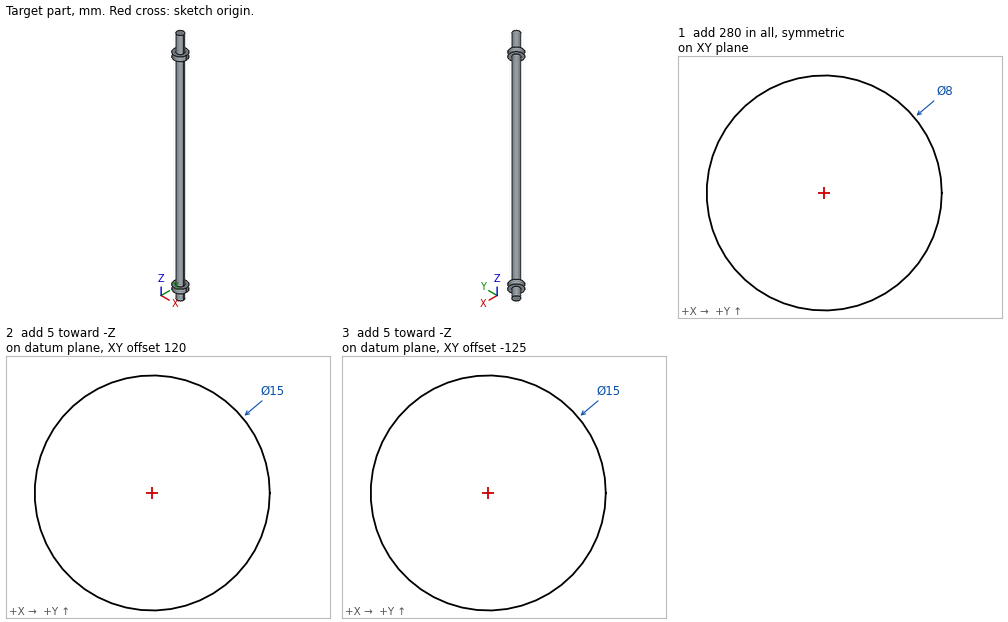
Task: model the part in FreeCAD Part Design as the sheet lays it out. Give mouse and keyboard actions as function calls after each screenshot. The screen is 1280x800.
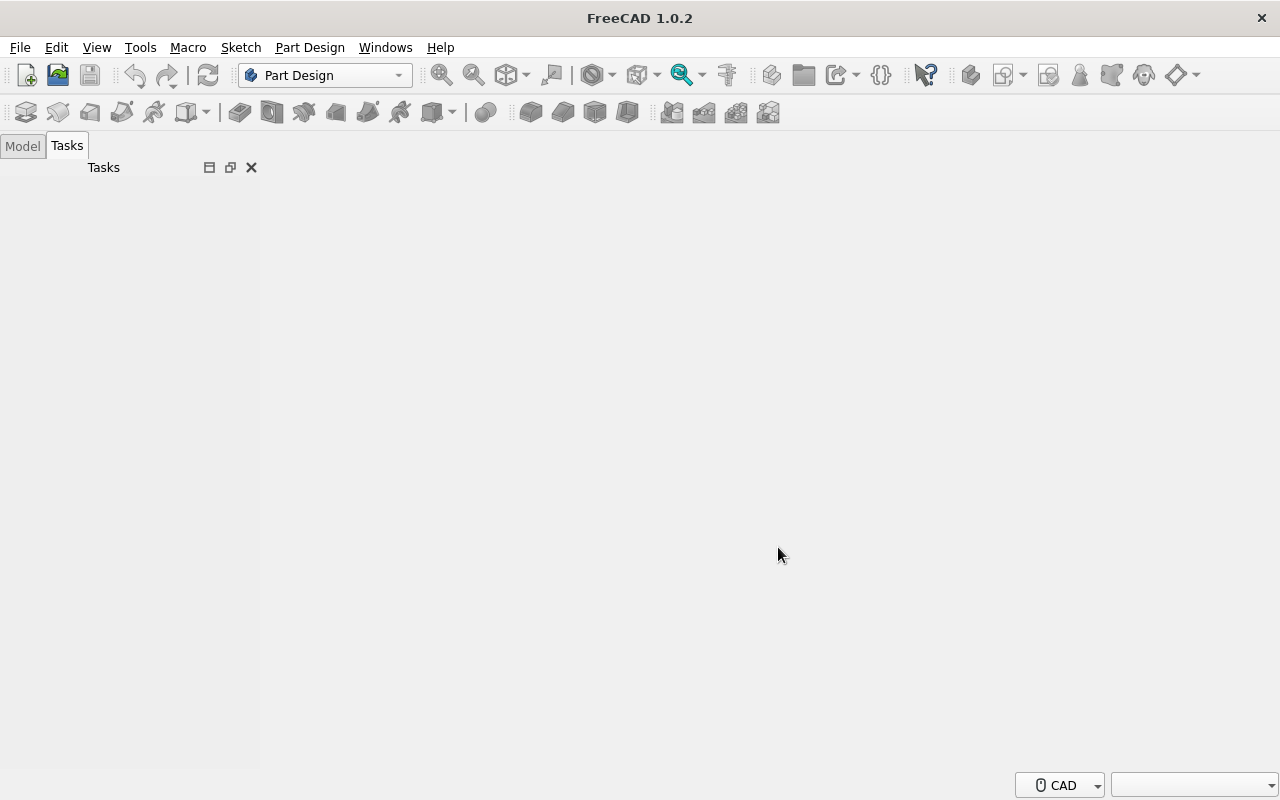
key(ctrl+n)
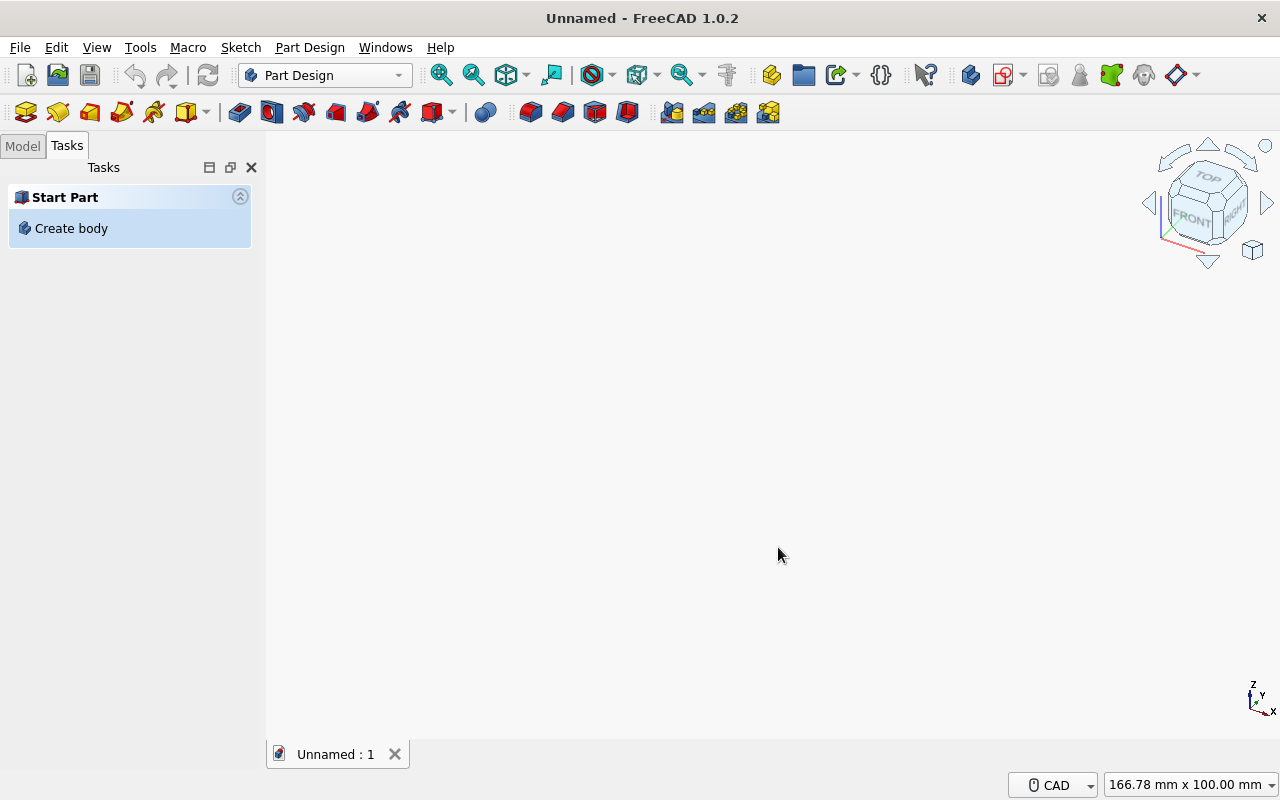
click(1004, 76)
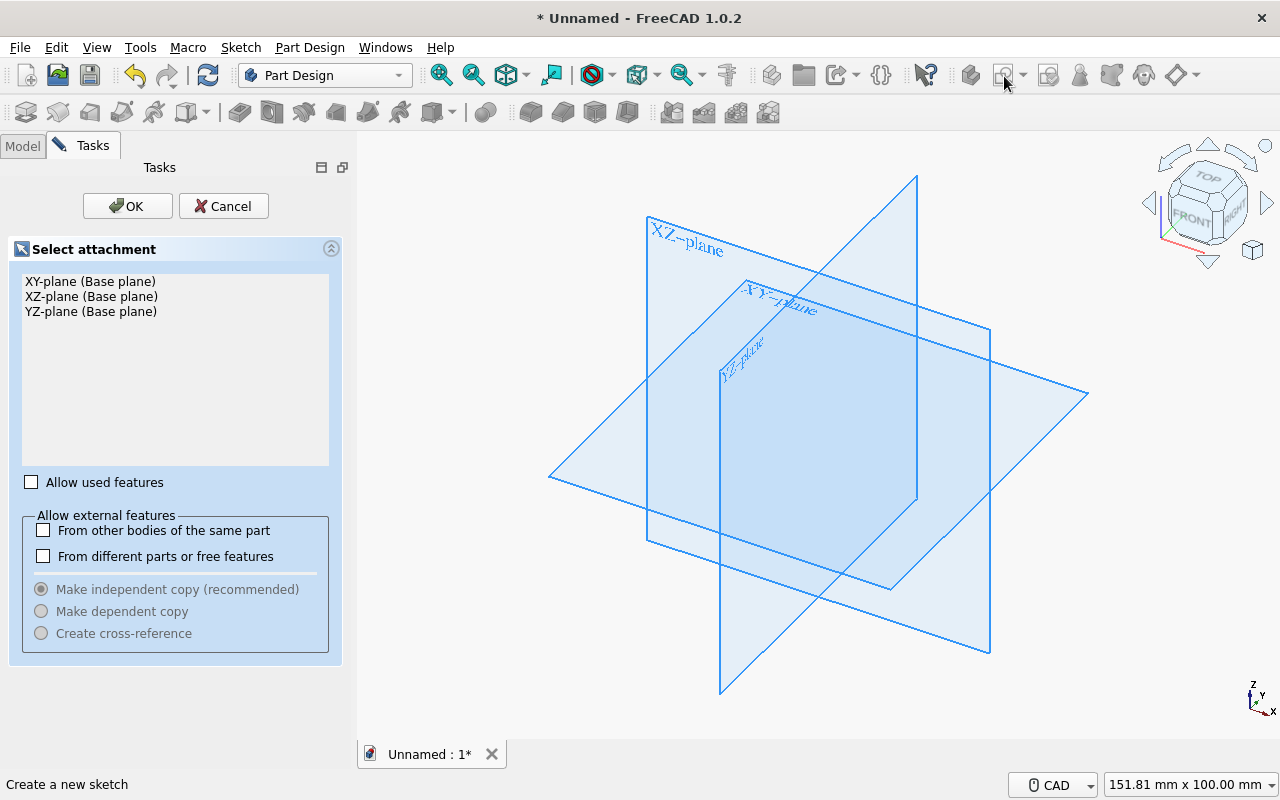
click(82, 282)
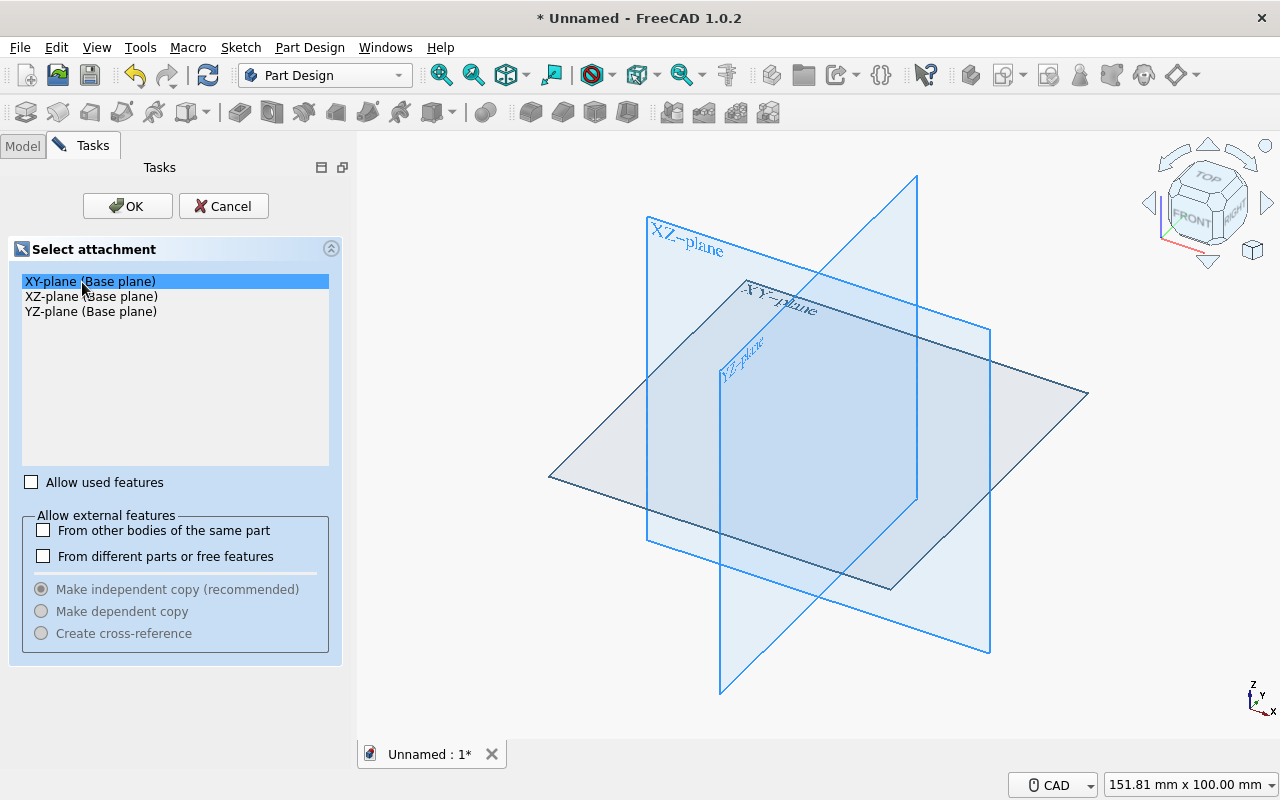
click(128, 206)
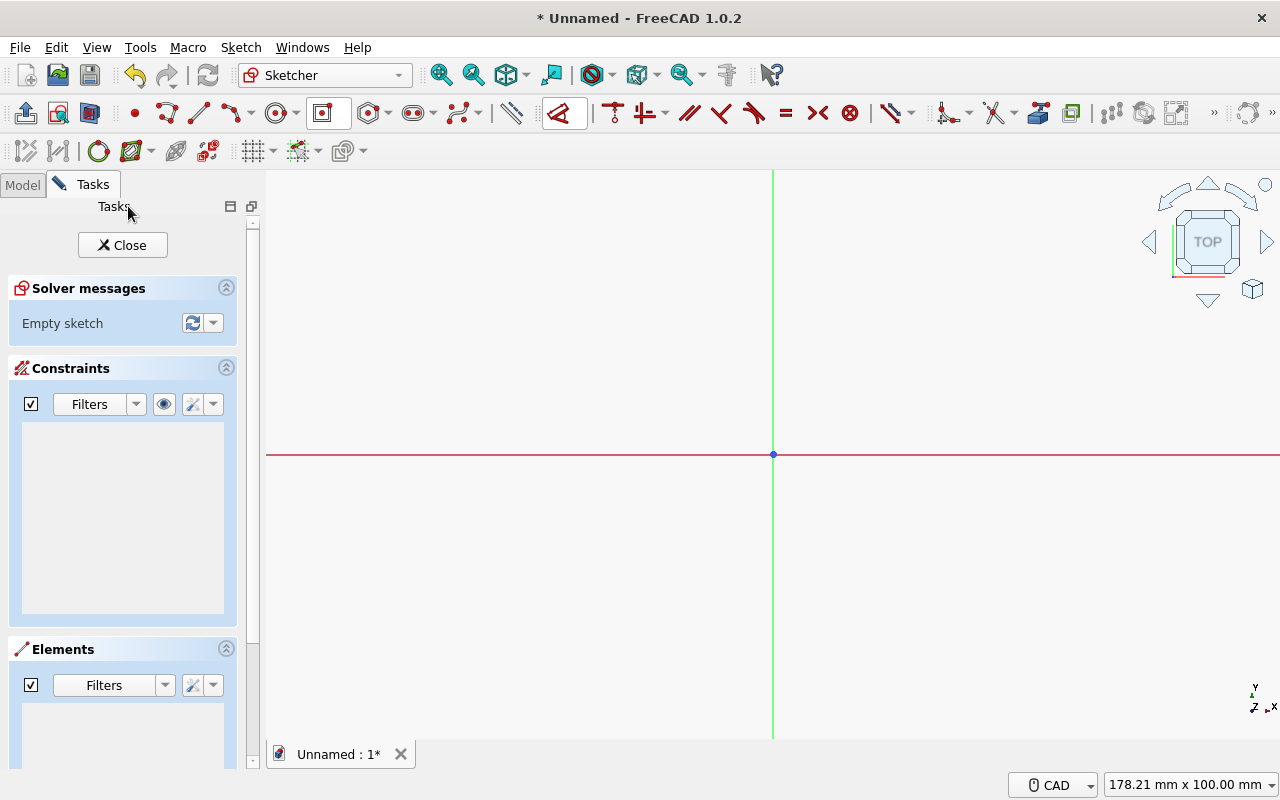
scroll(784, 454, up, 10)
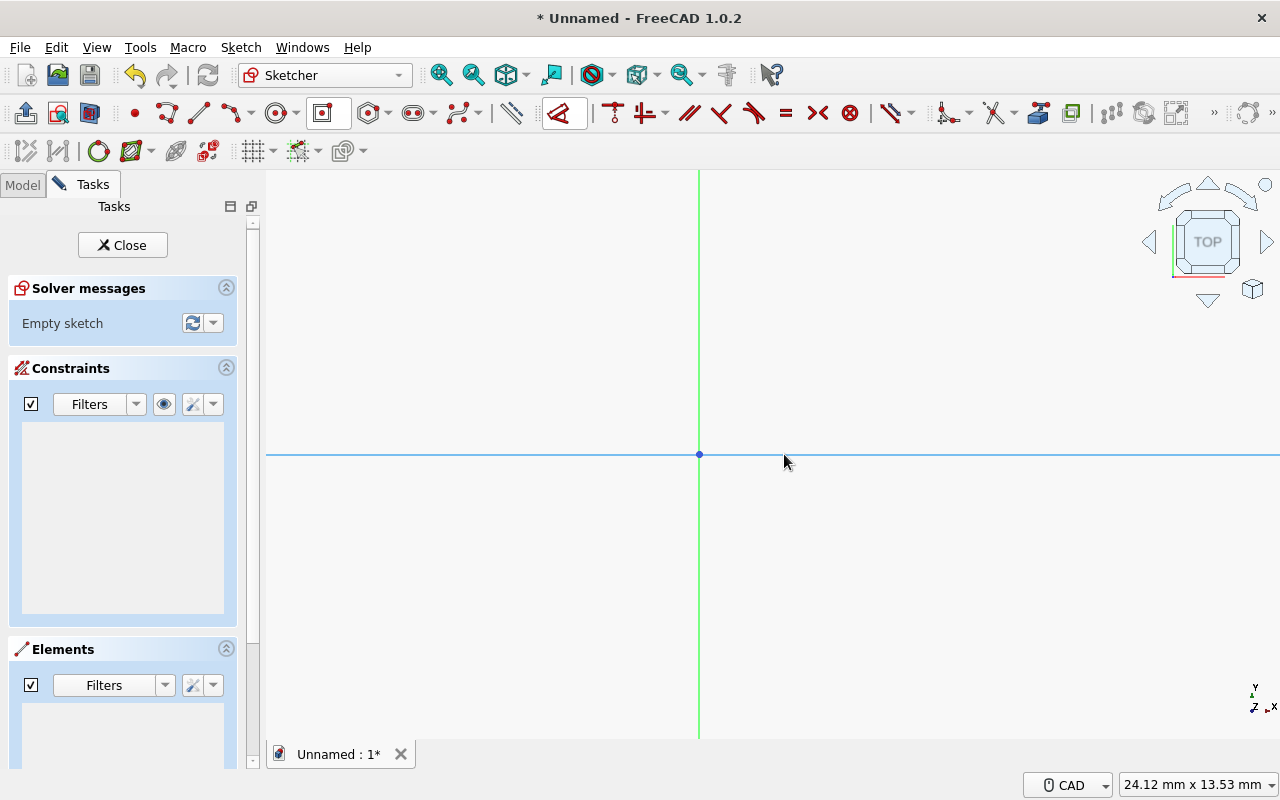
key(g)
key(c)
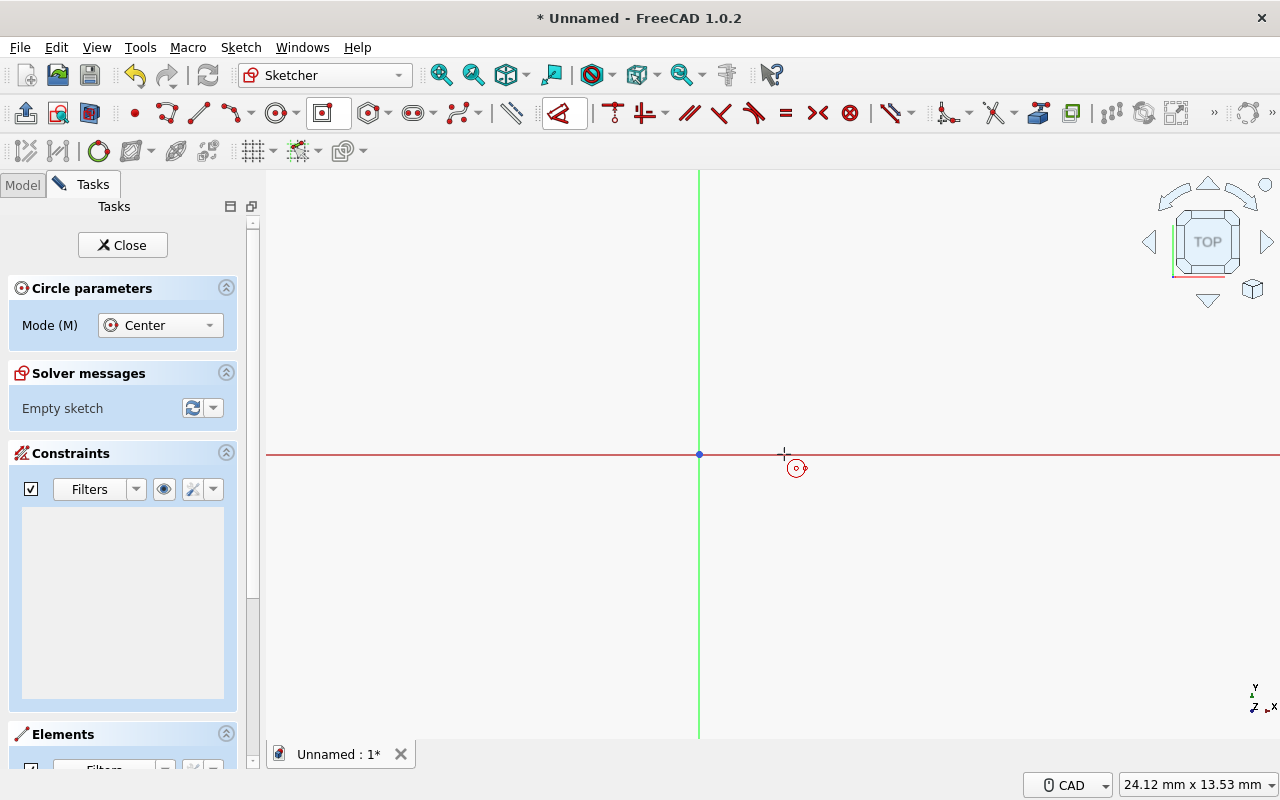
click(699, 454)
click(818, 336)
key(Escape)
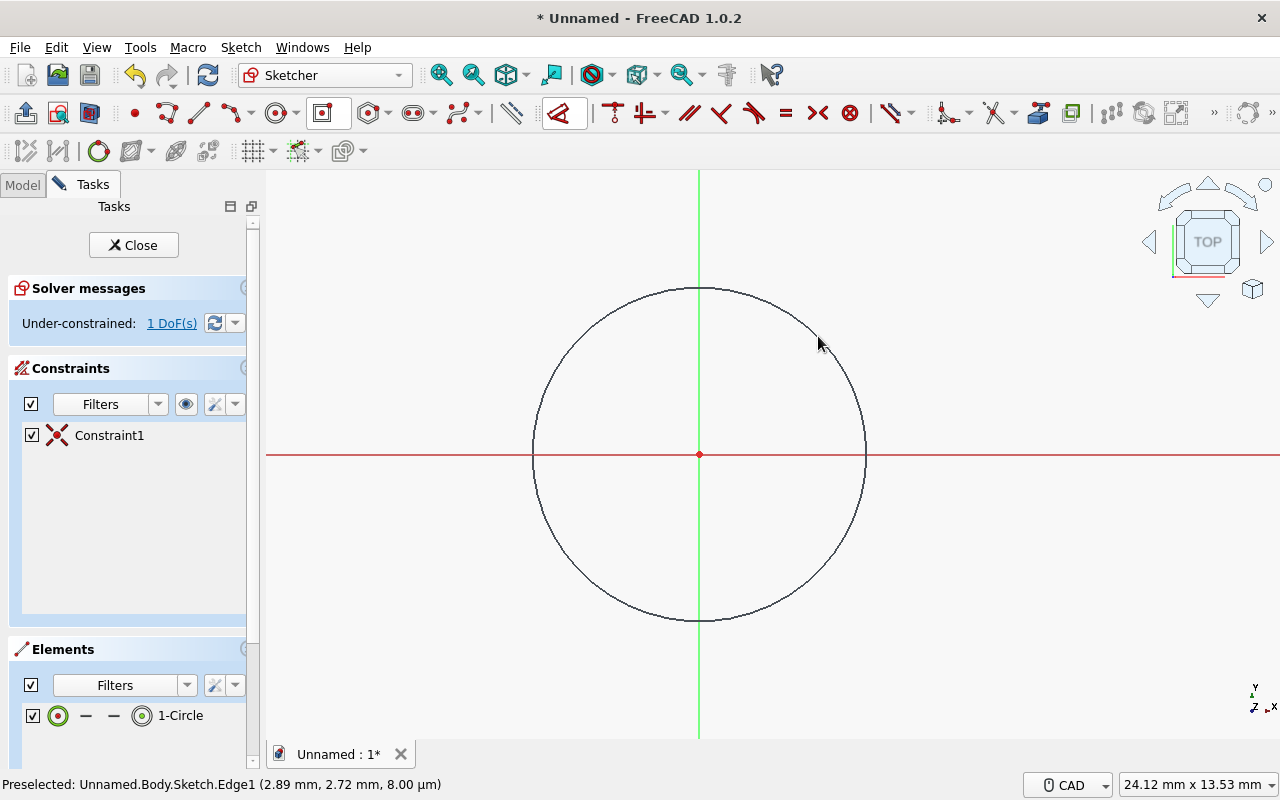
click(817, 336)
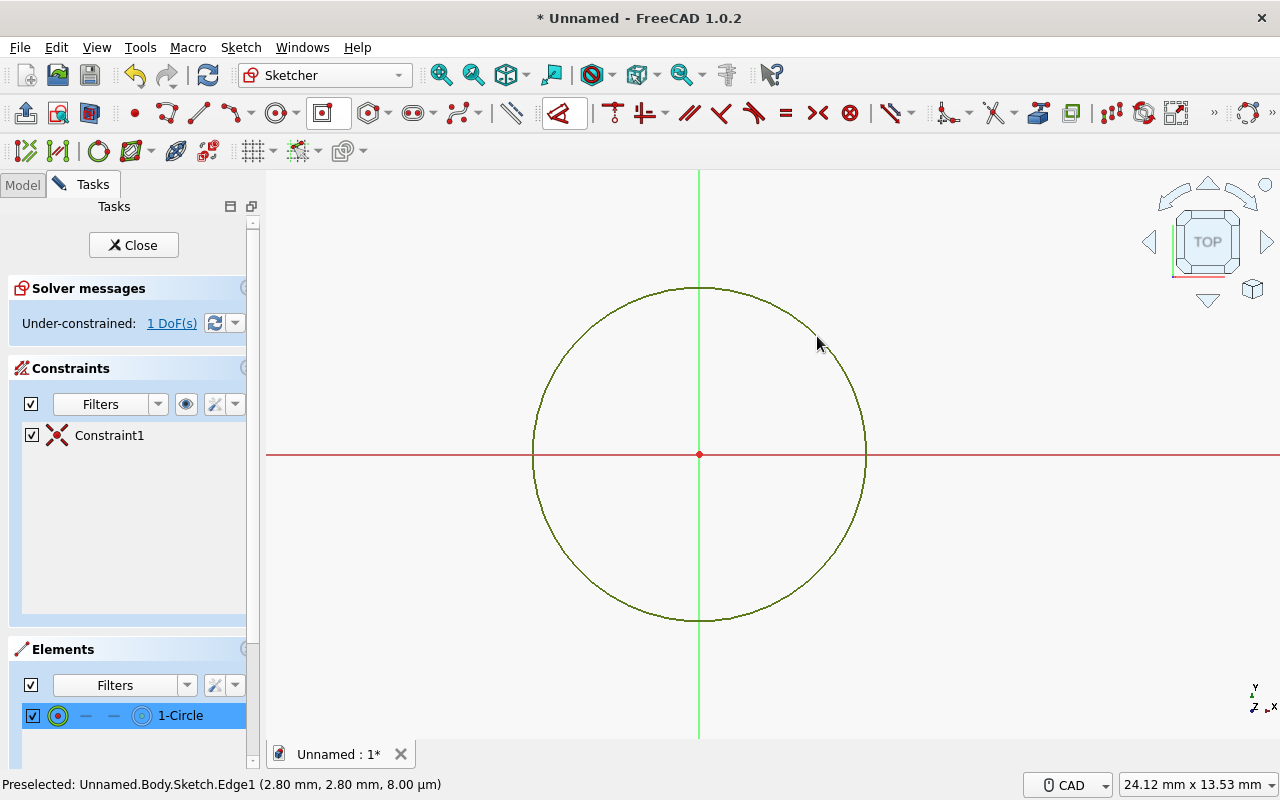
key(k)
key(o)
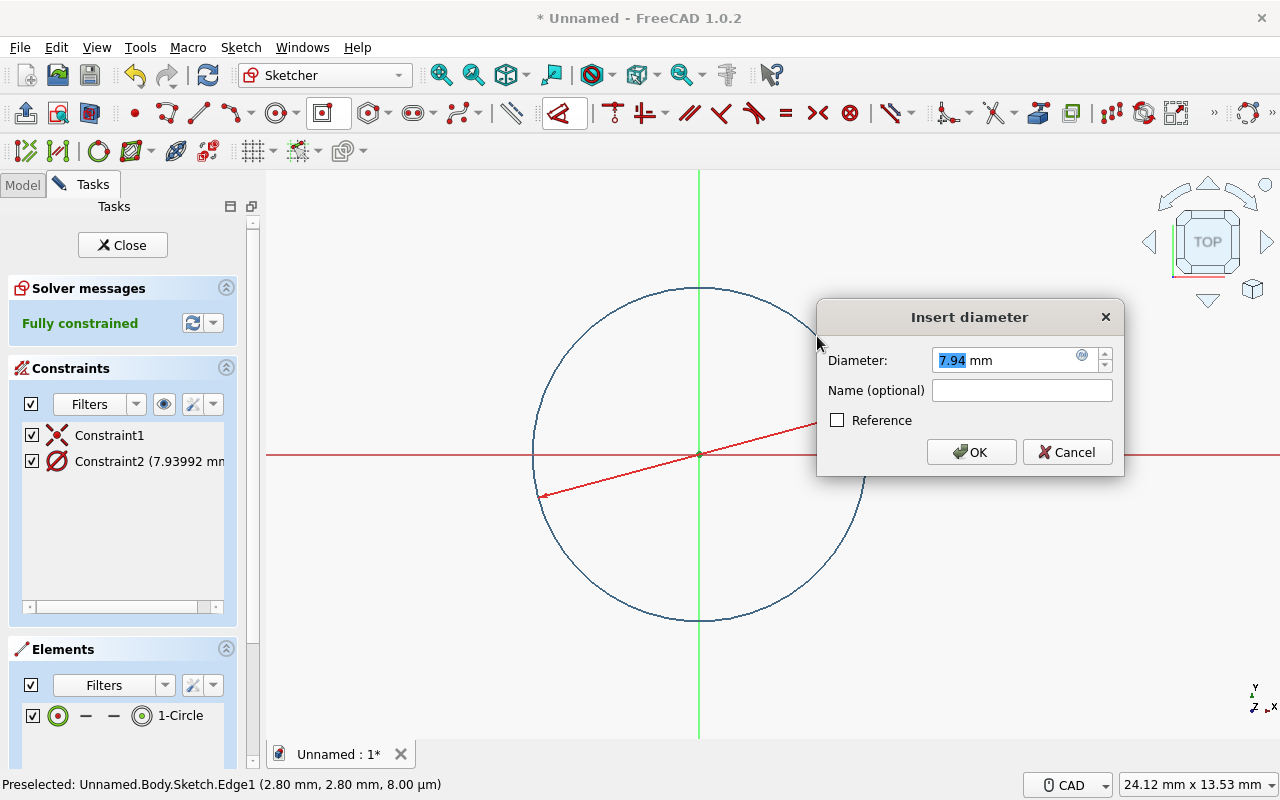
text(8)
key(Return)